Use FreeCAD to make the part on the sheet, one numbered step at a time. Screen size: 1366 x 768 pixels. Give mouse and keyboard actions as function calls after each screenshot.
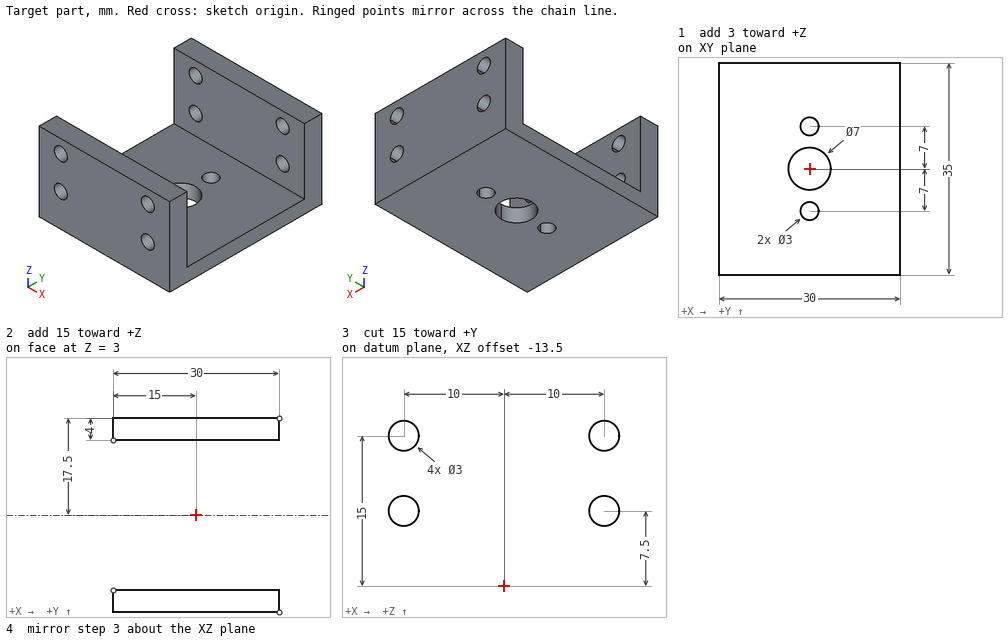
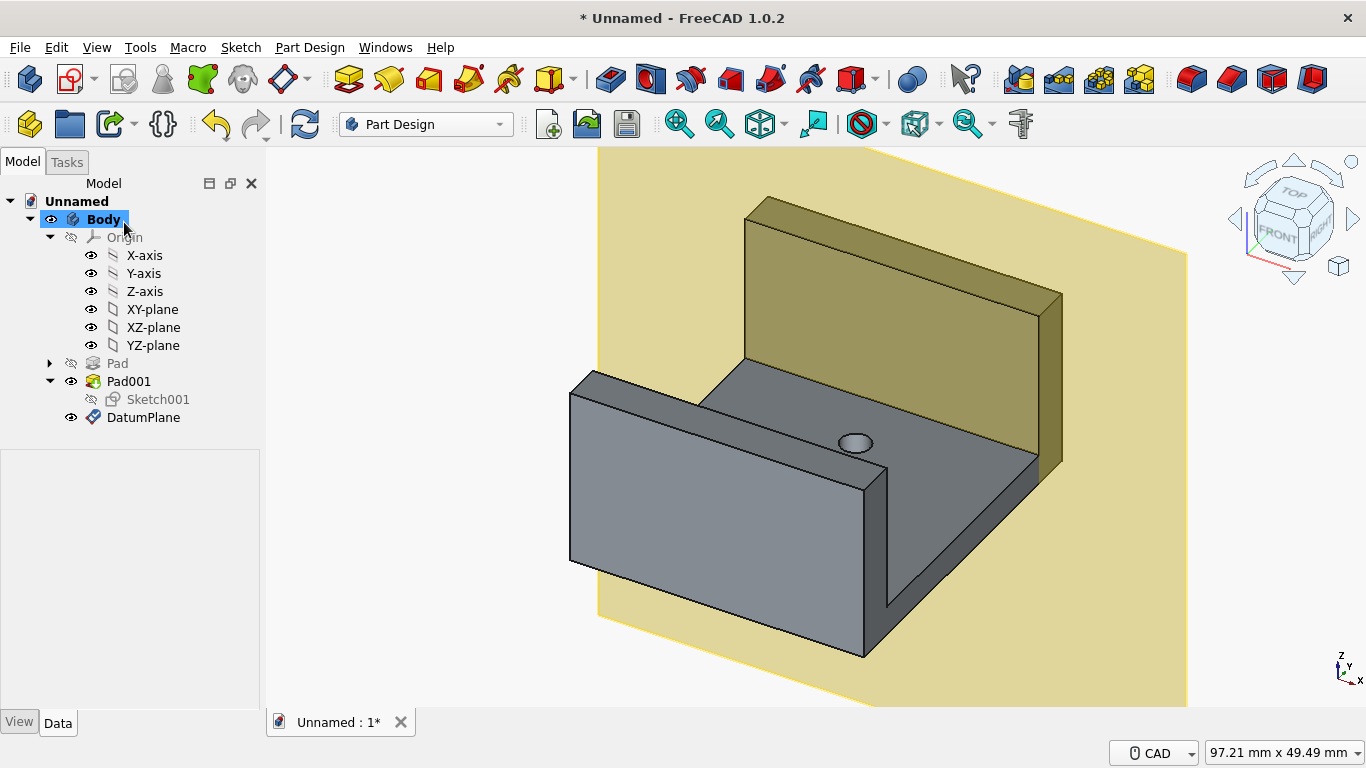
click(116, 417)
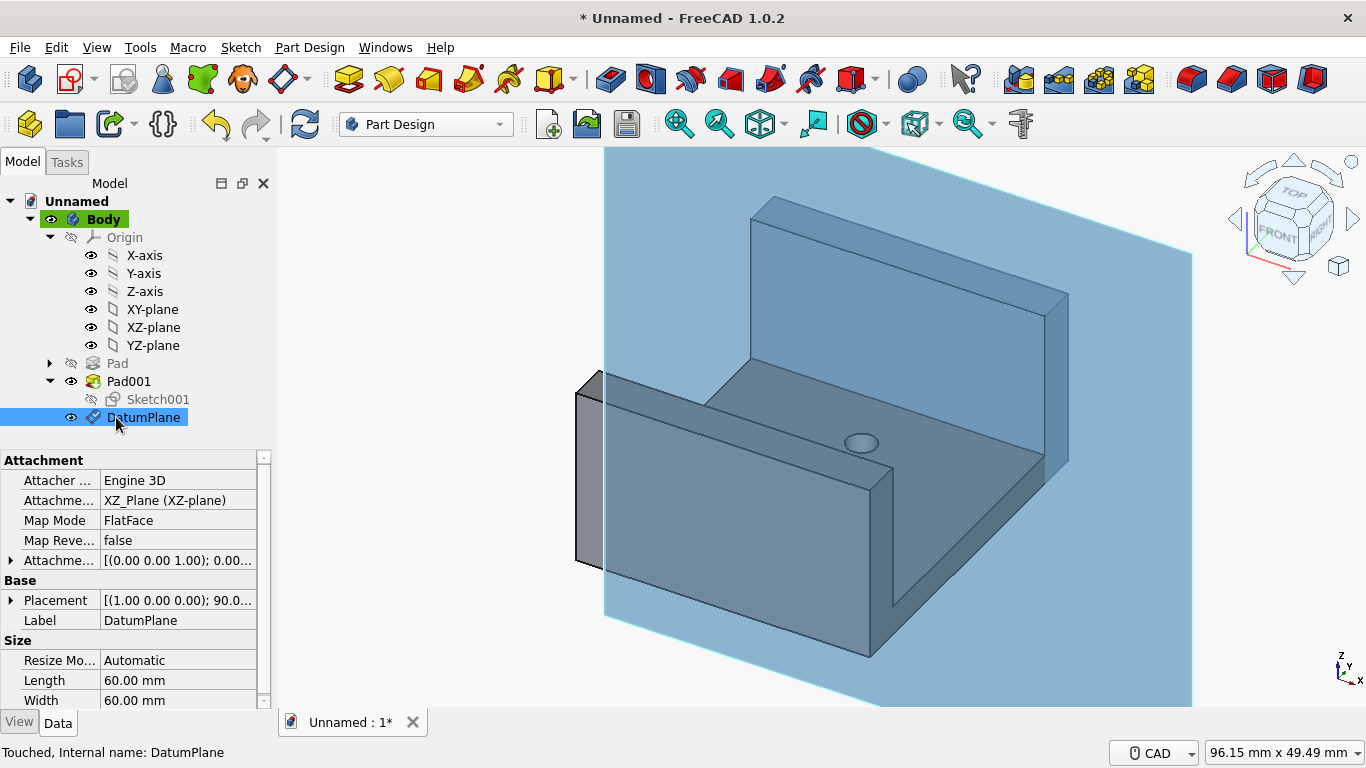
click(70, 80)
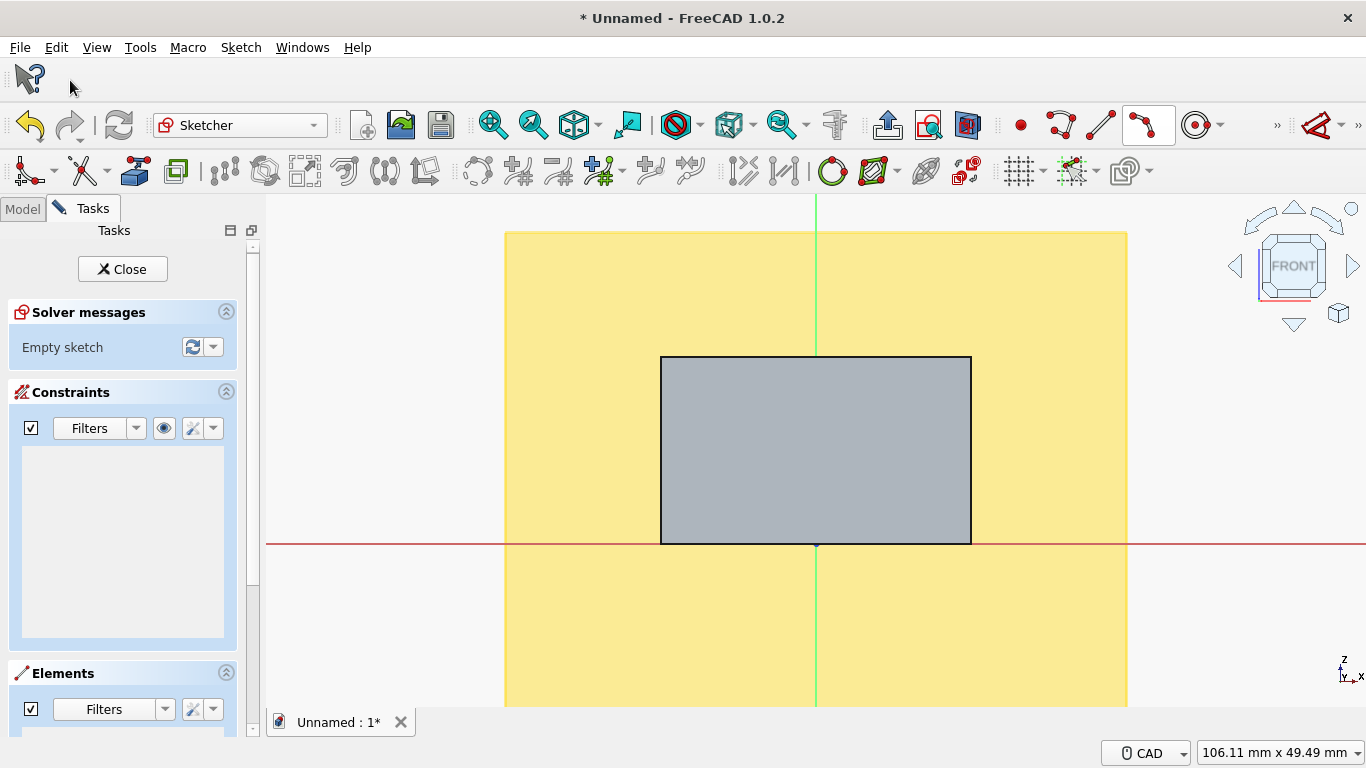
click(968, 126)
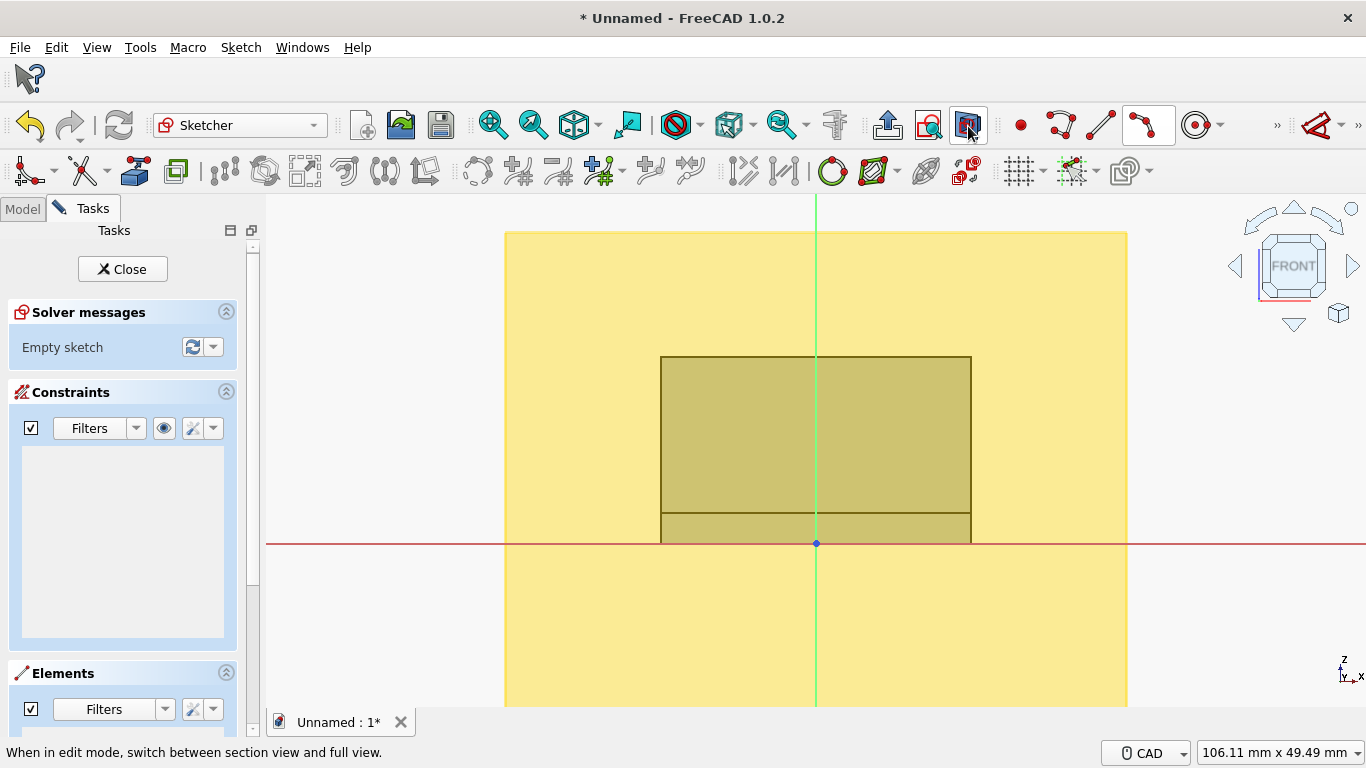
scroll(899, 468, up, 3)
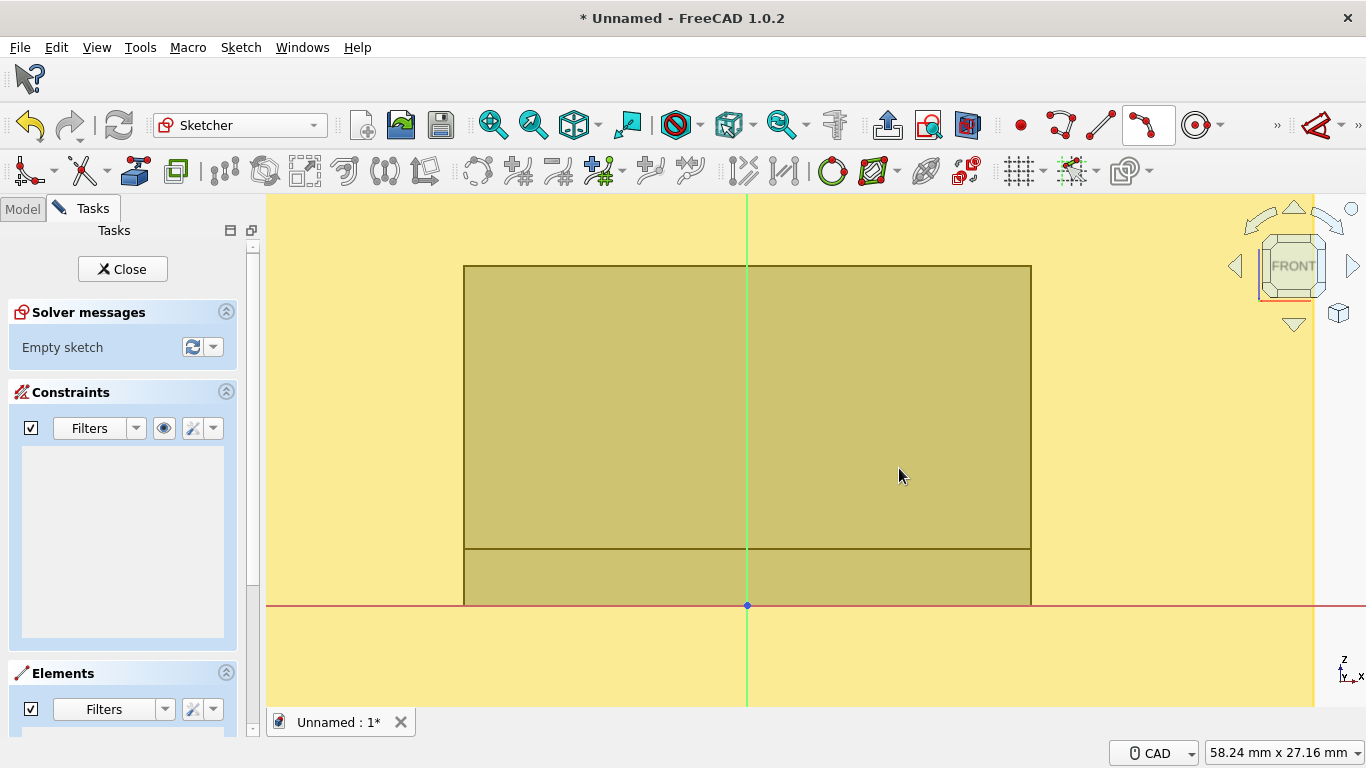
click(1196, 126)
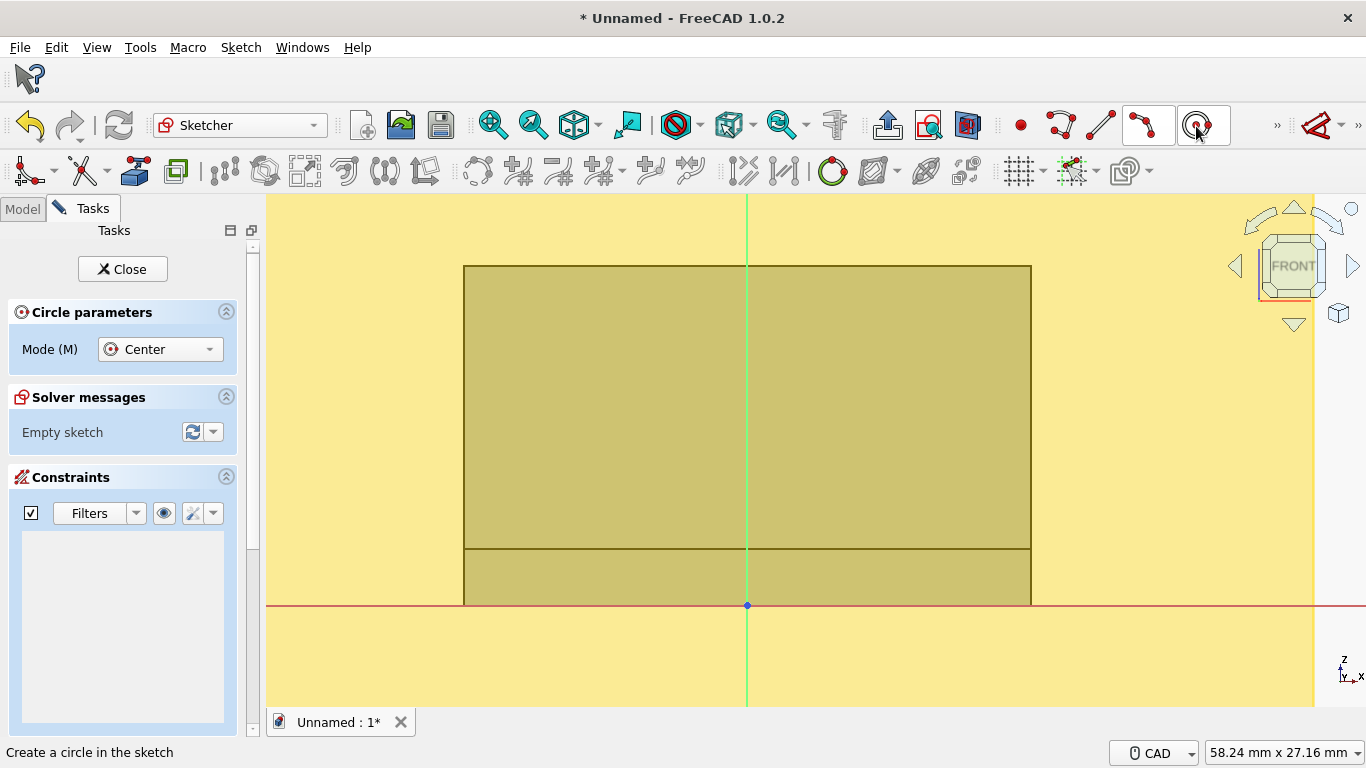
click(558, 322)
click(578, 302)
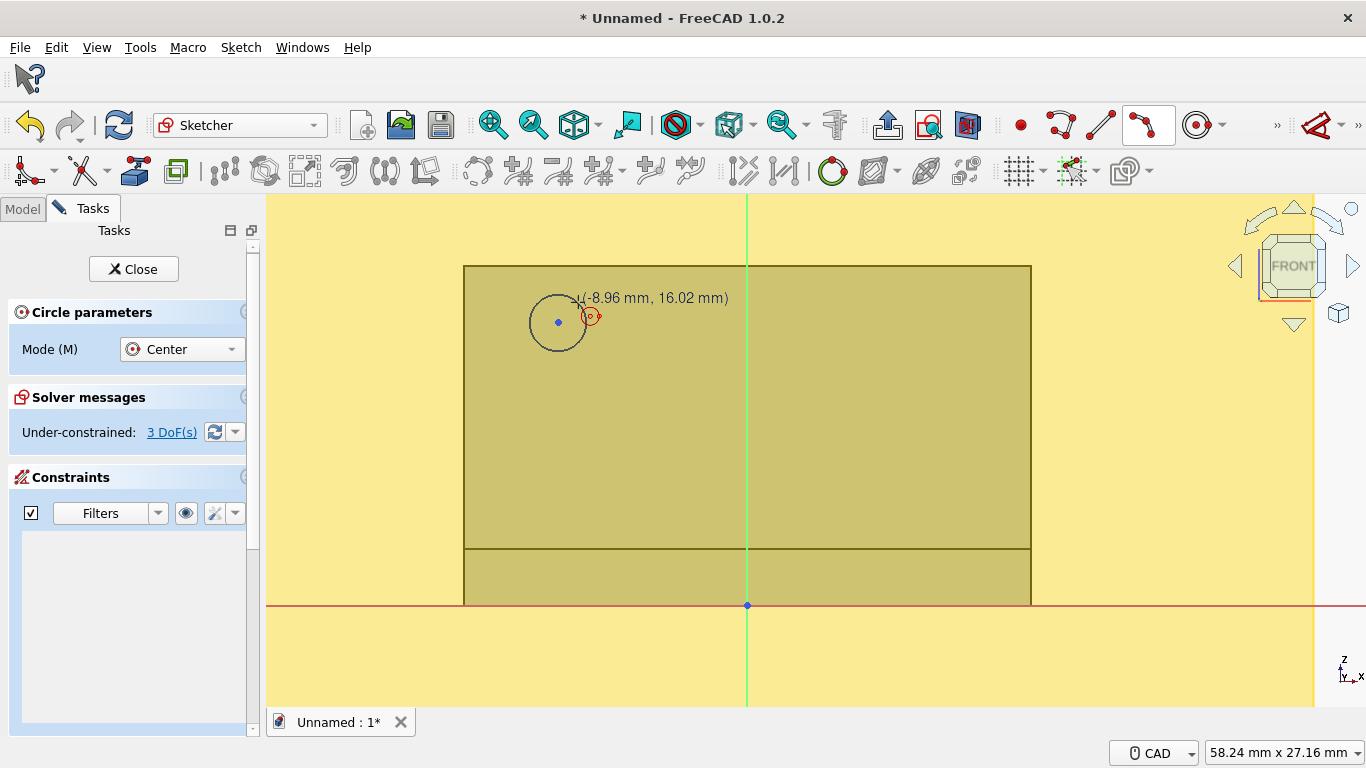
click(936, 322)
click(956, 302)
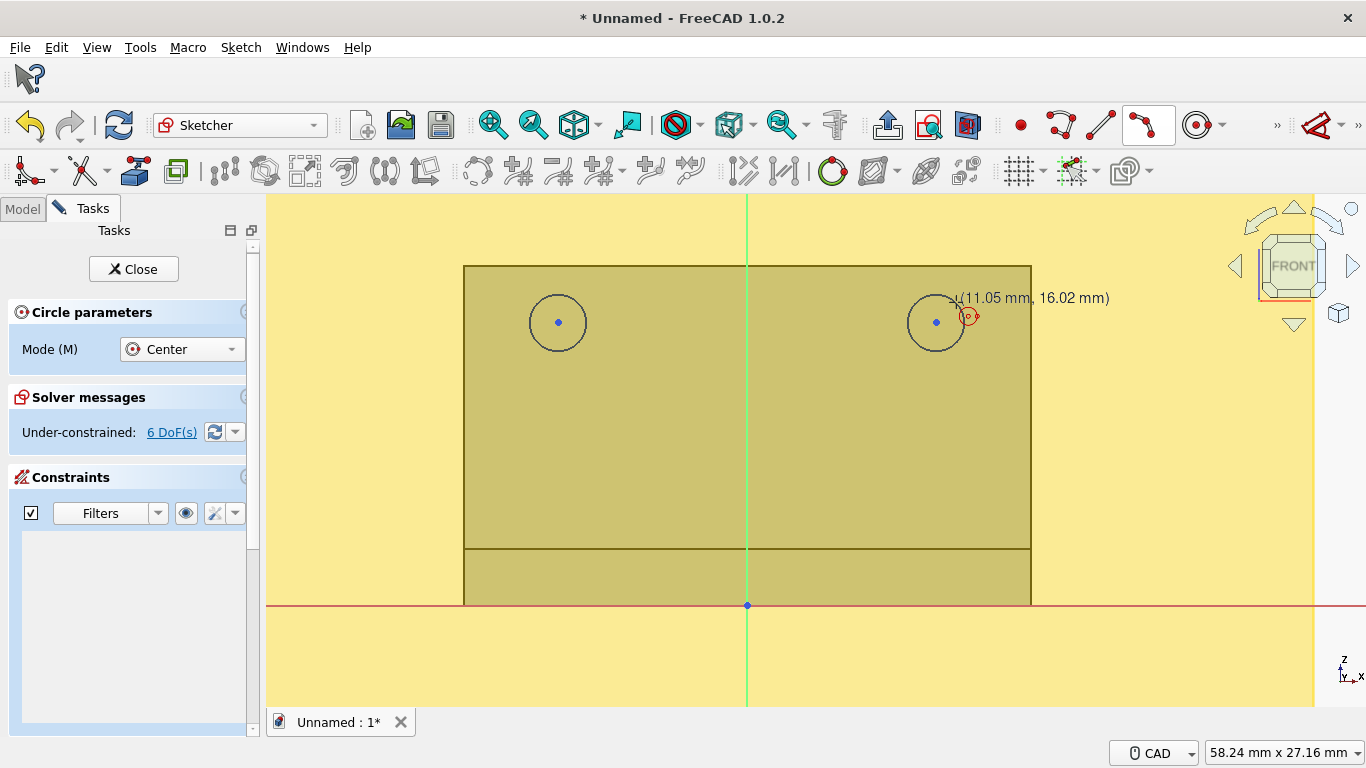
click(936, 464)
click(956, 444)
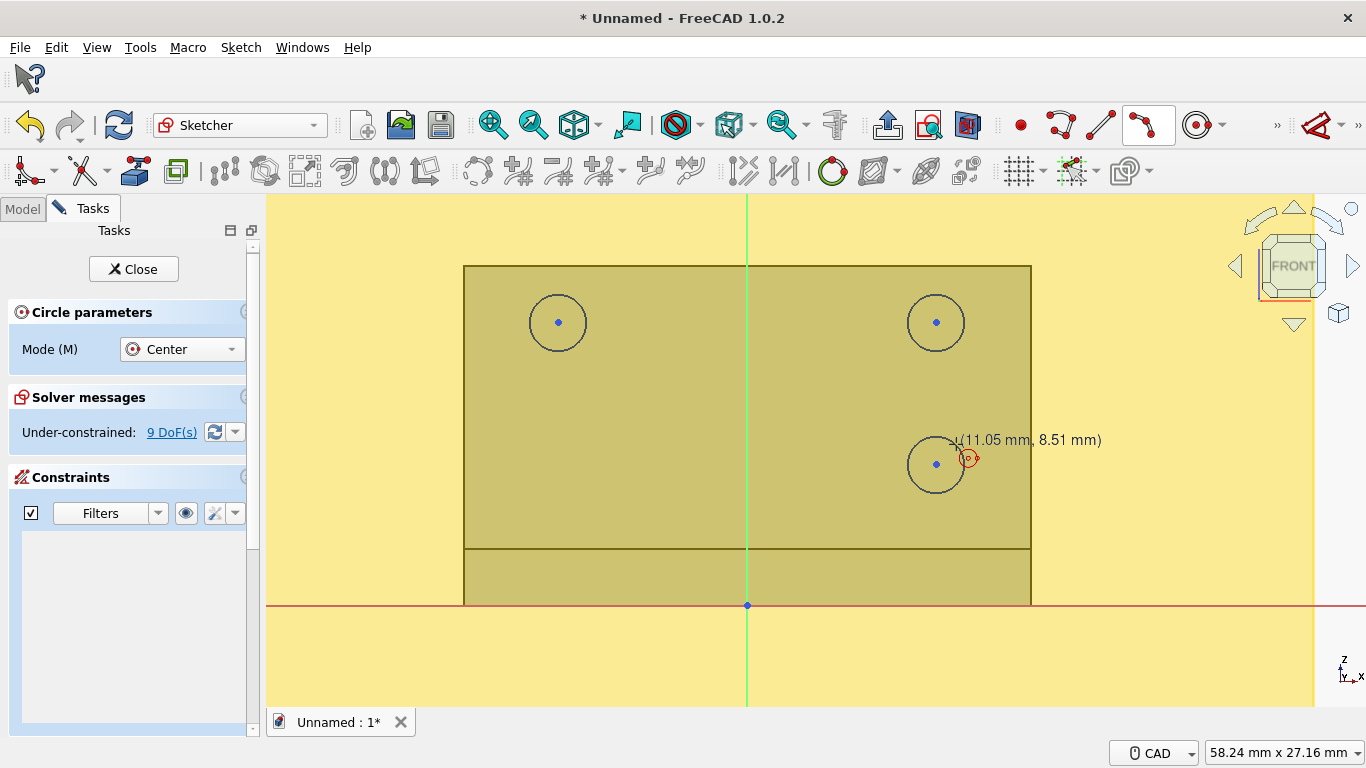
click(558, 464)
click(578, 444)
key(Escape)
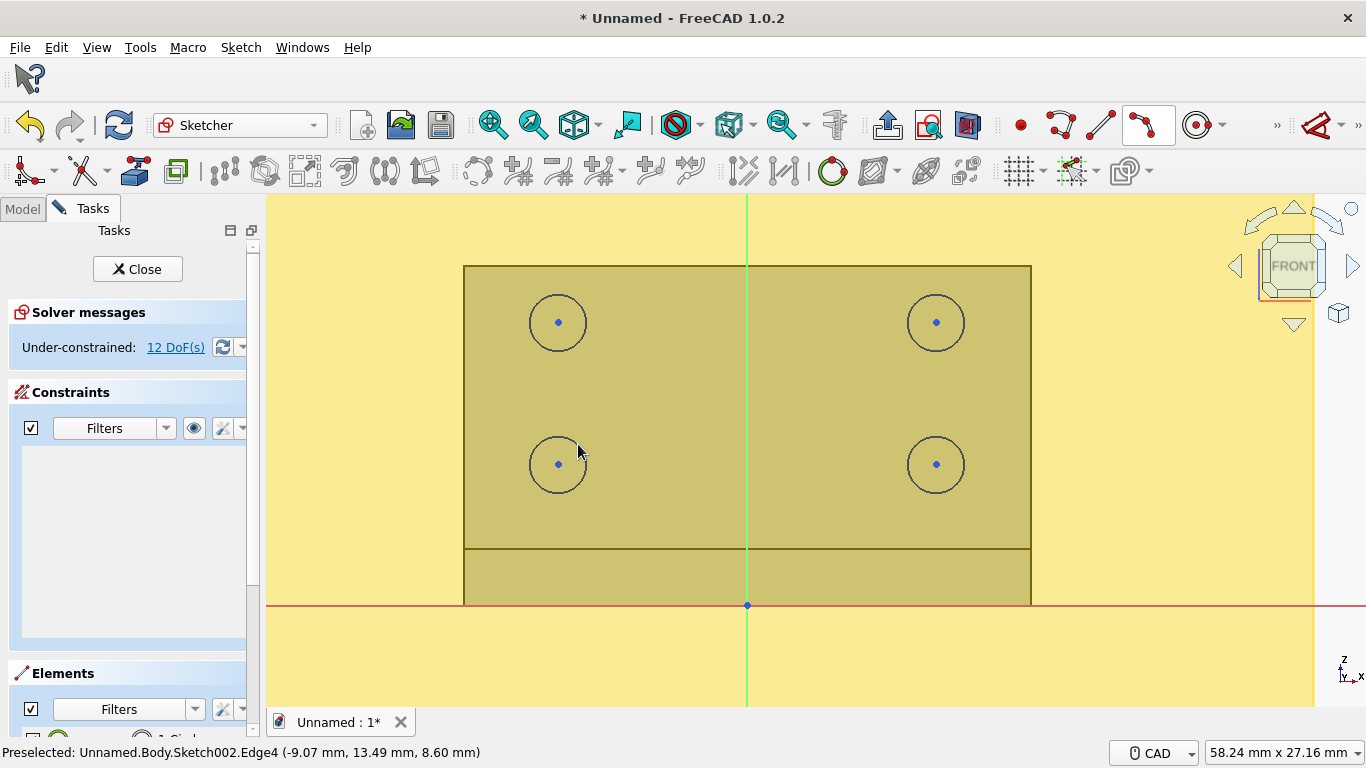
click(578, 303)